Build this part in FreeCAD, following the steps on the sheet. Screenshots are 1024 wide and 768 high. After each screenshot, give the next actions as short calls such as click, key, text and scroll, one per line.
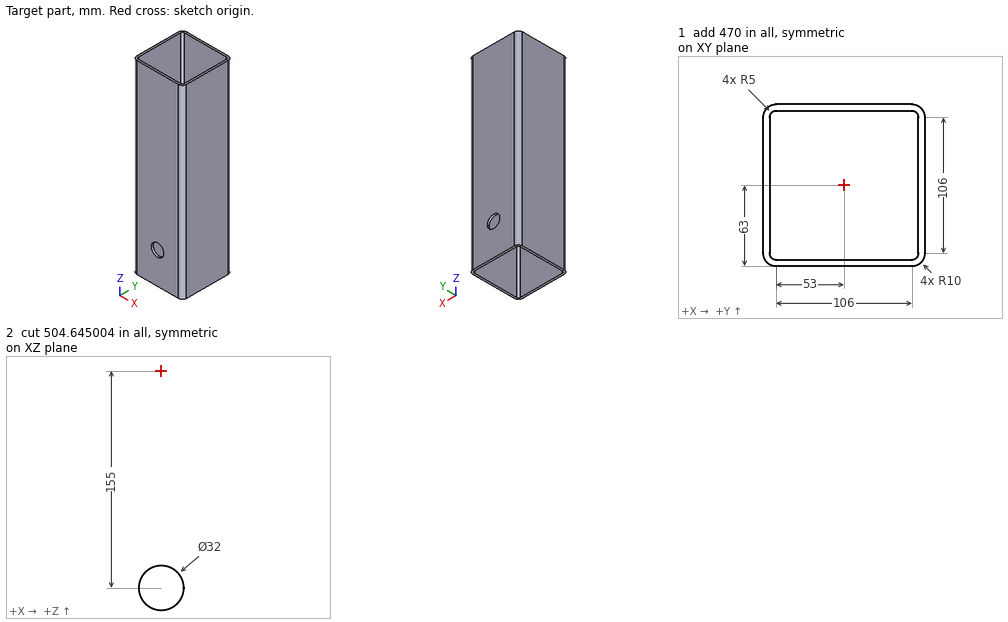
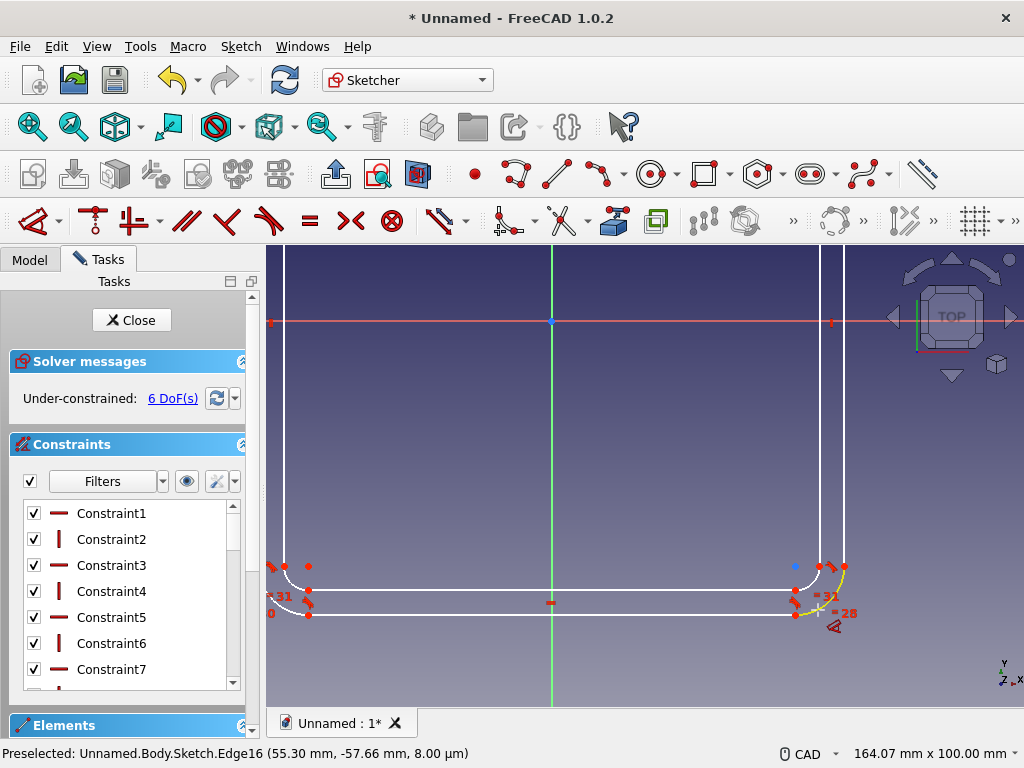
click(818, 610)
click(833, 638)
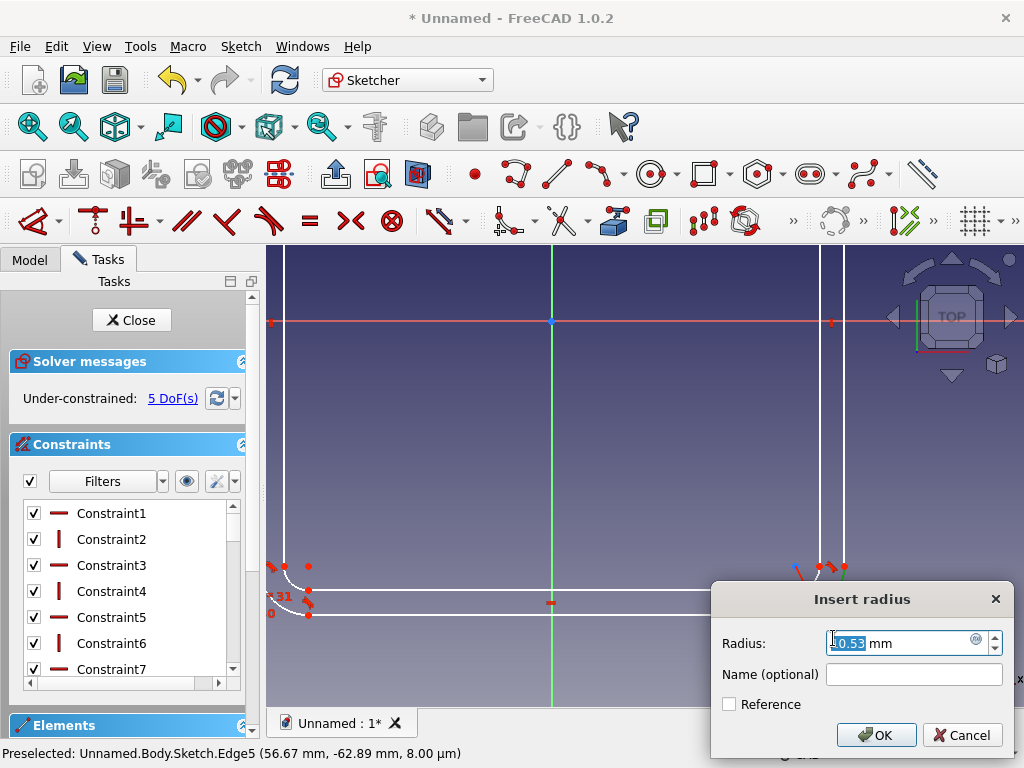
text(10)
key(Return)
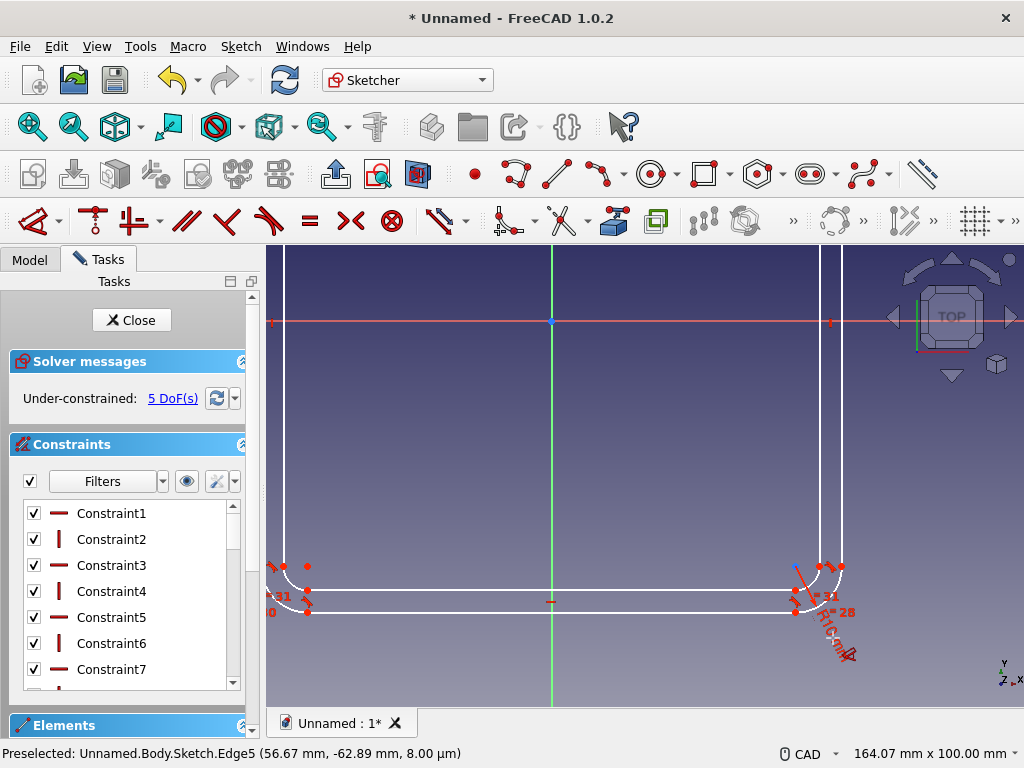
scroll(297, 588, up, 3)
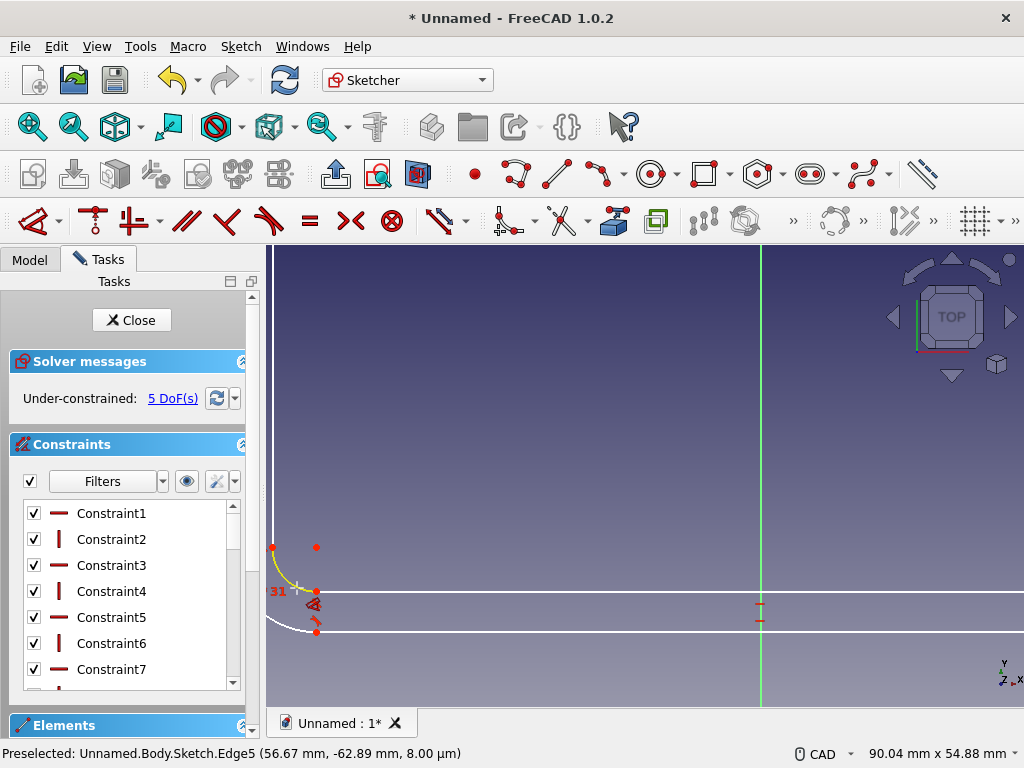
click(296, 587)
click(354, 614)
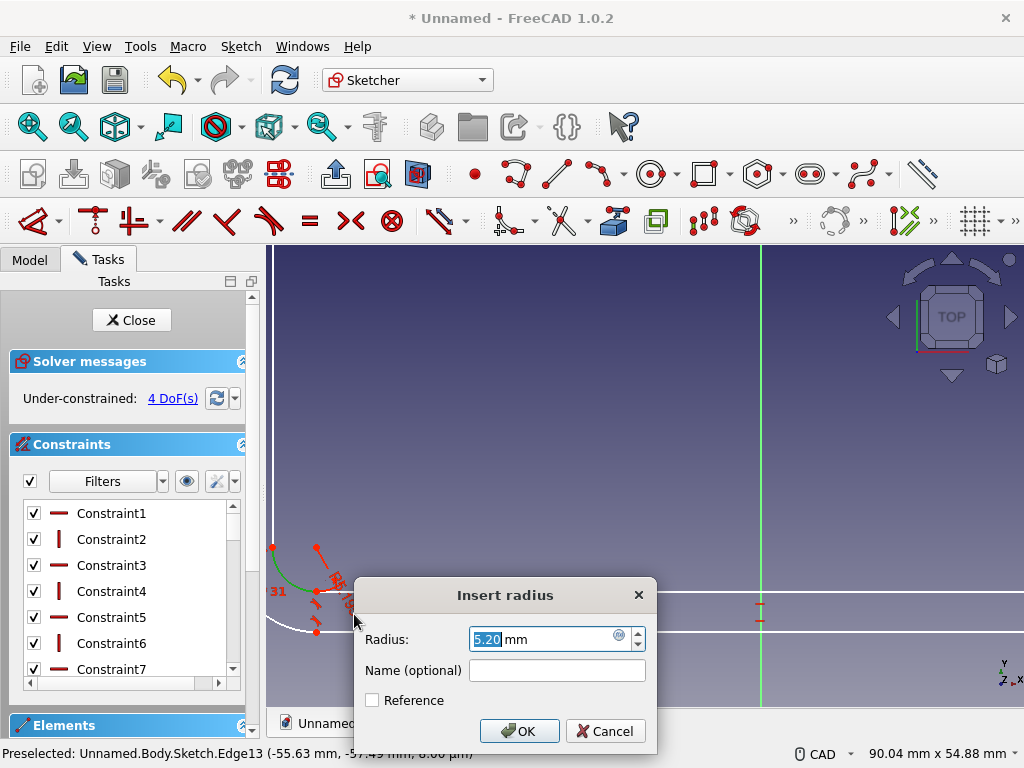
text(5)
key(Return)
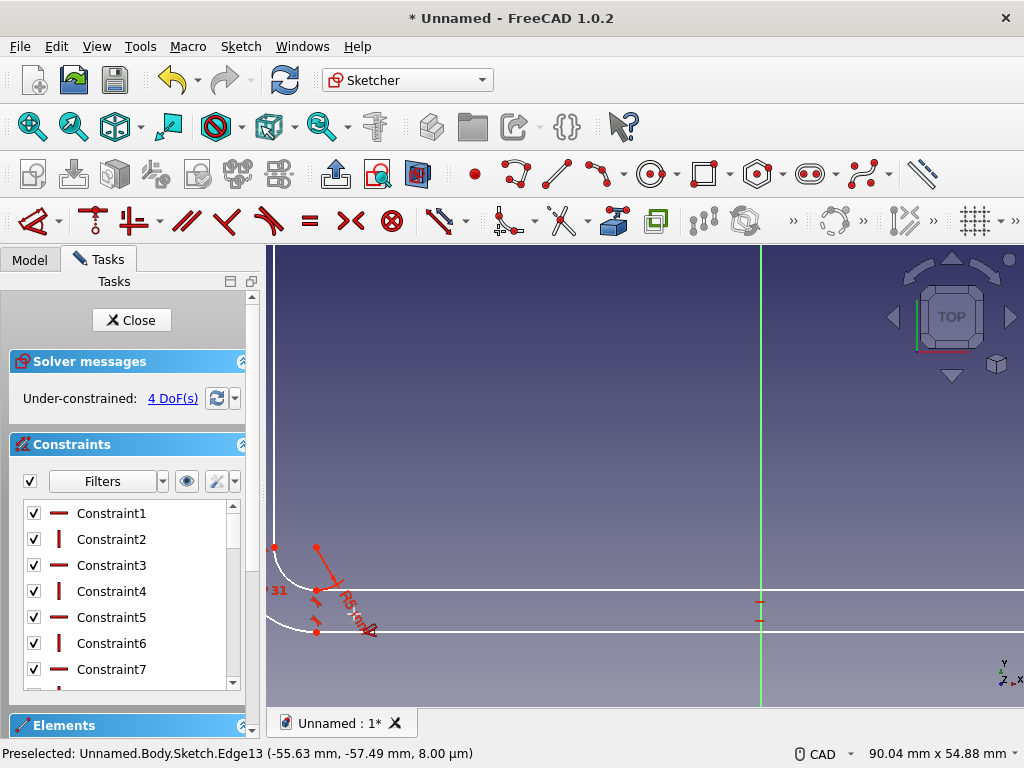
scroll(516, 599, down, 7)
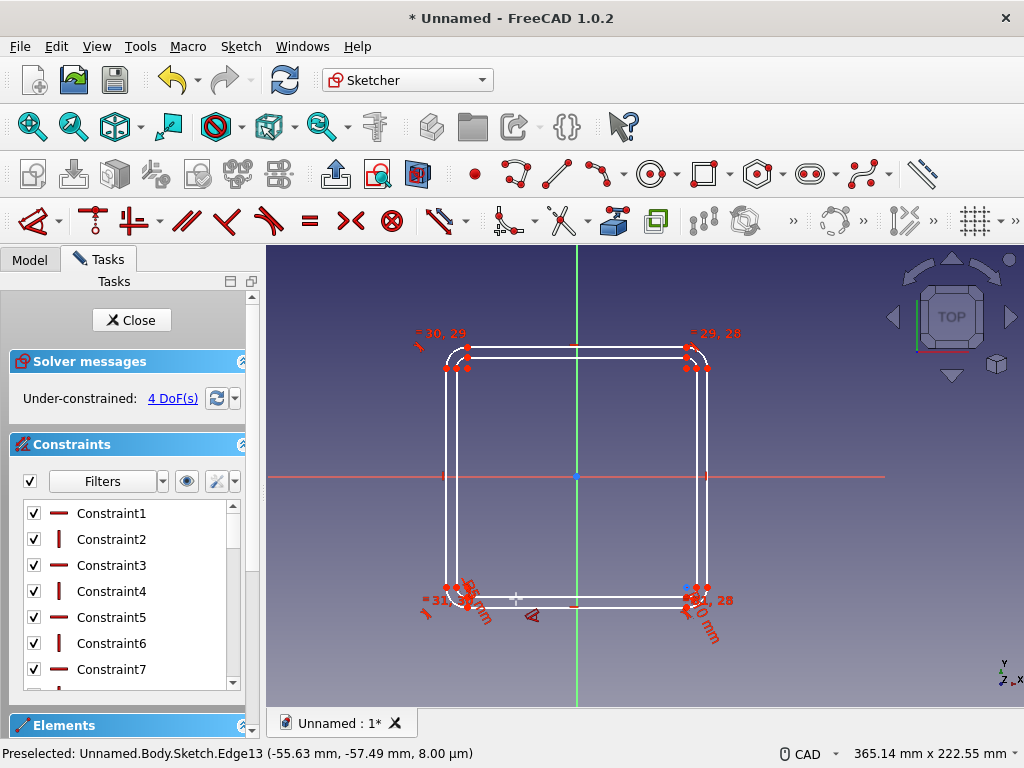
scroll(533, 608, up, 2)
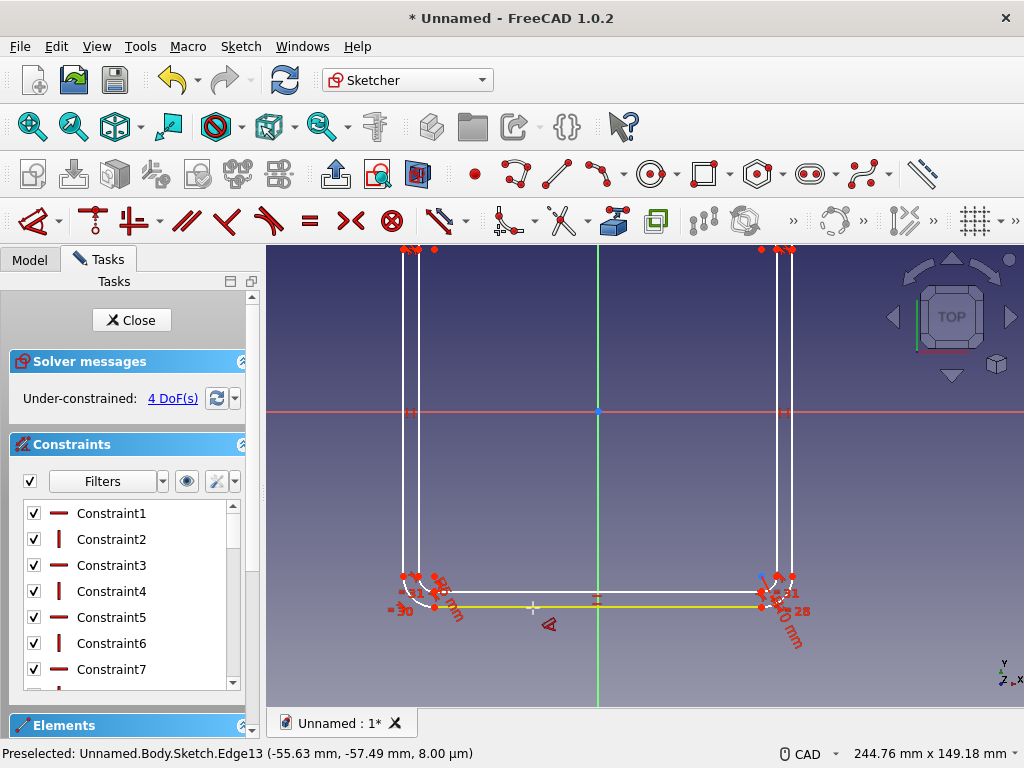
click(533, 607)
click(523, 641)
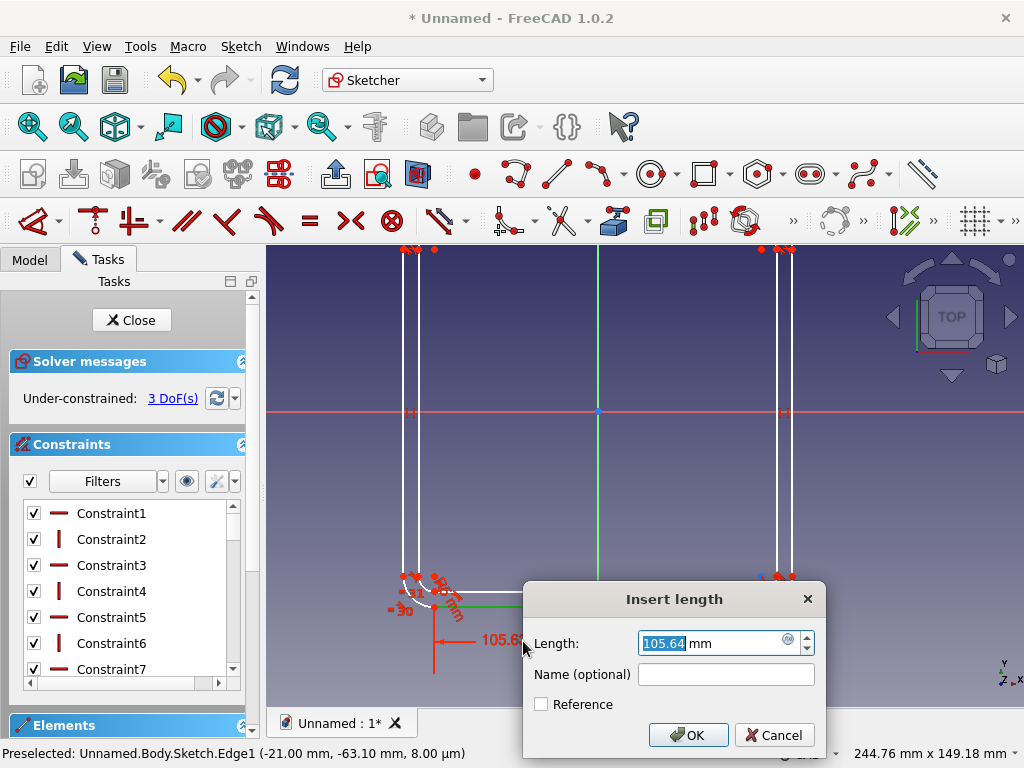
text(106)
key(Return)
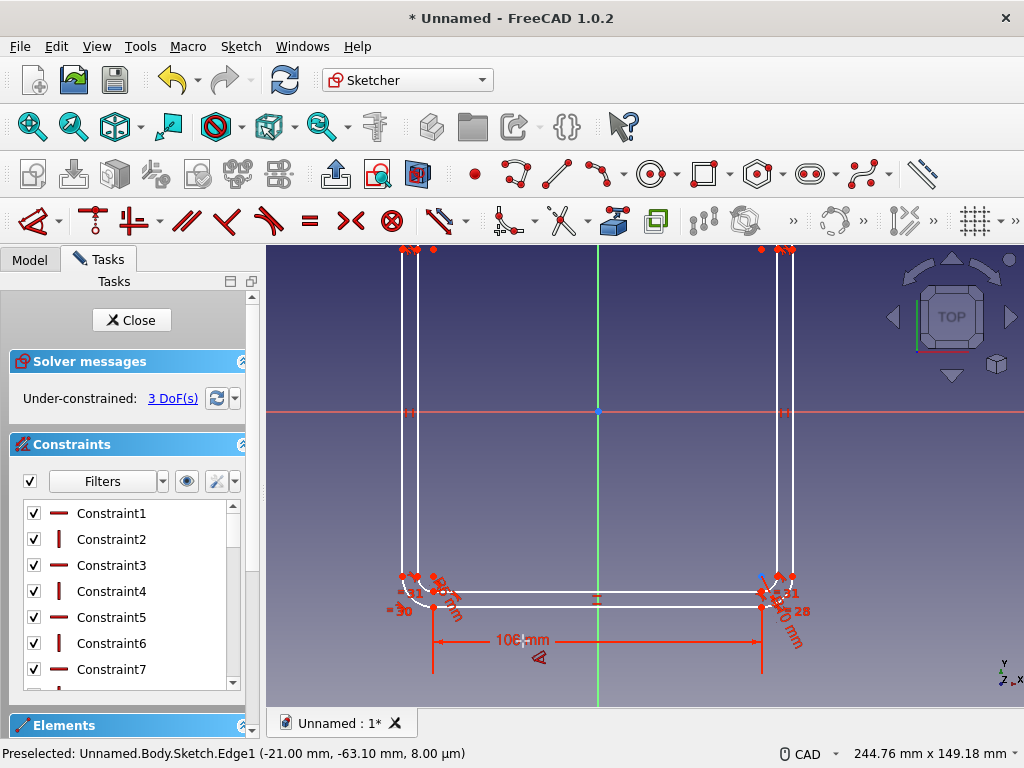
click(793, 478)
click(827, 355)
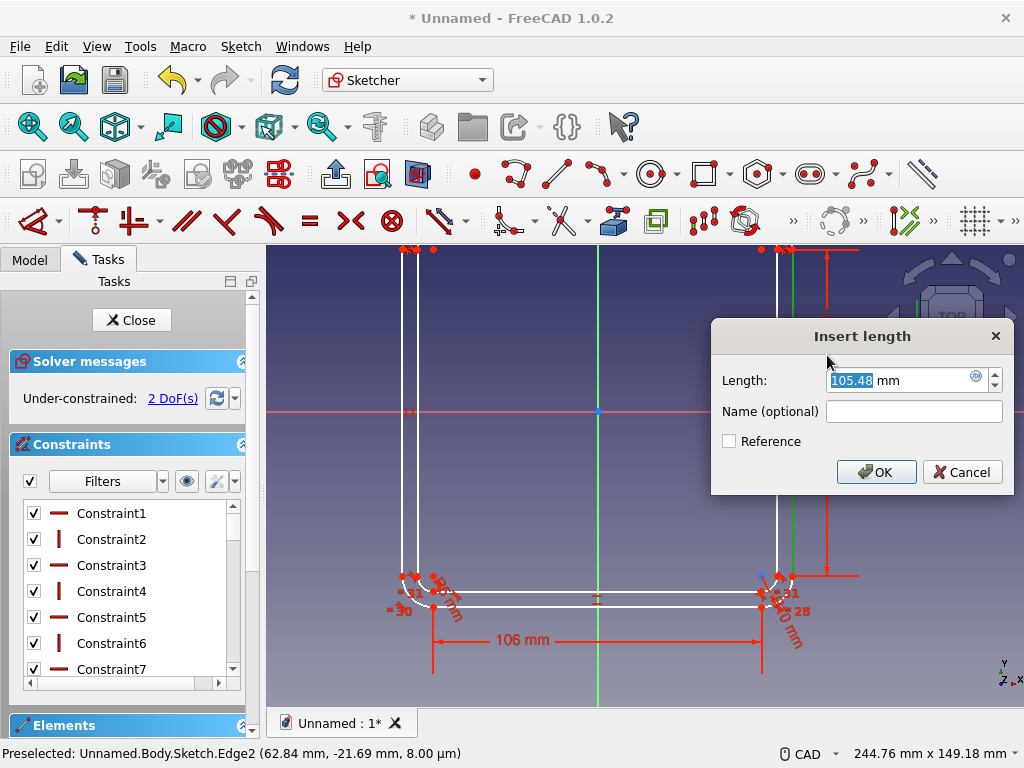
text(106)
key(Return)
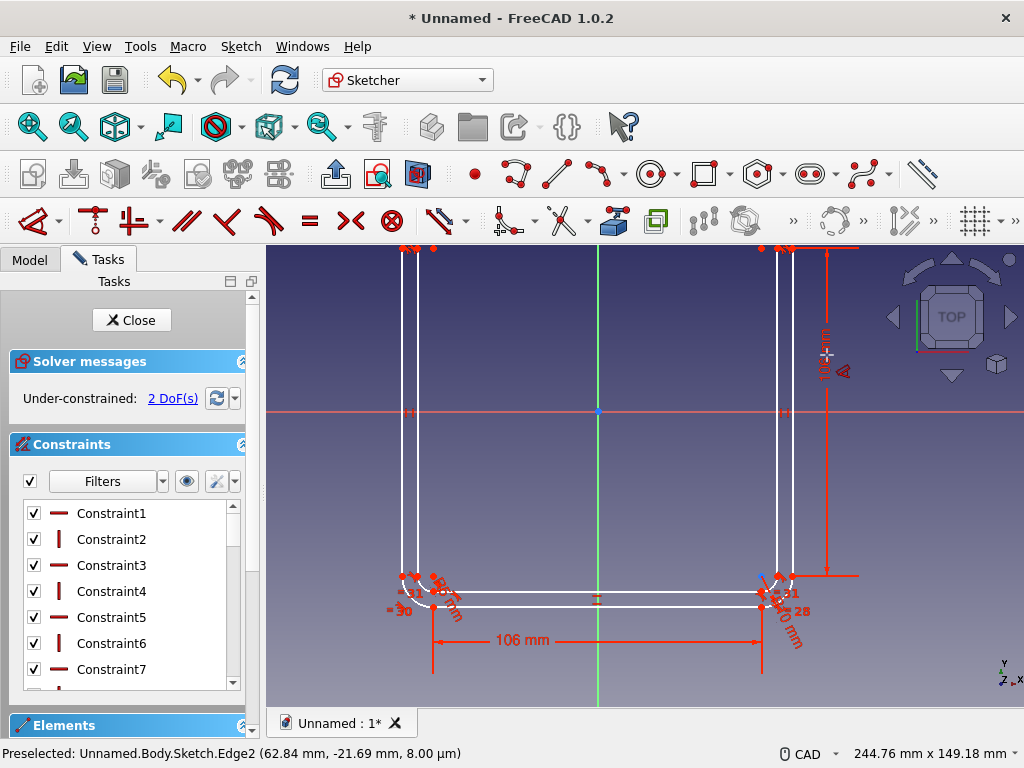
click(433, 607)
click(516, 378)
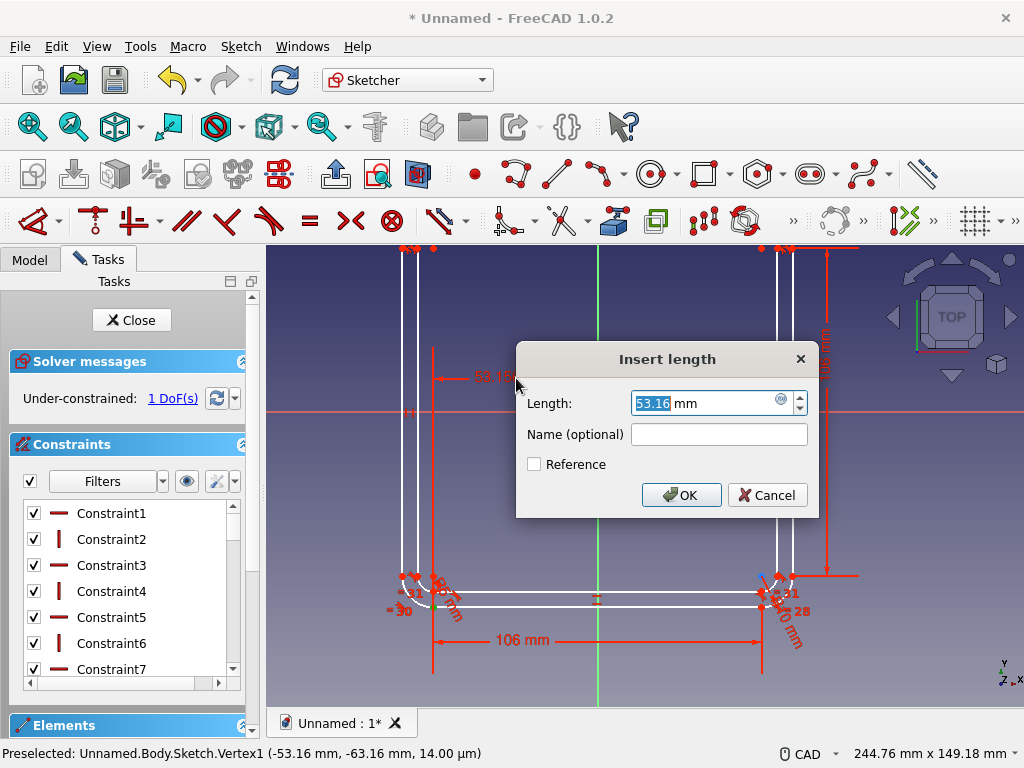
text(53)
key(Return)